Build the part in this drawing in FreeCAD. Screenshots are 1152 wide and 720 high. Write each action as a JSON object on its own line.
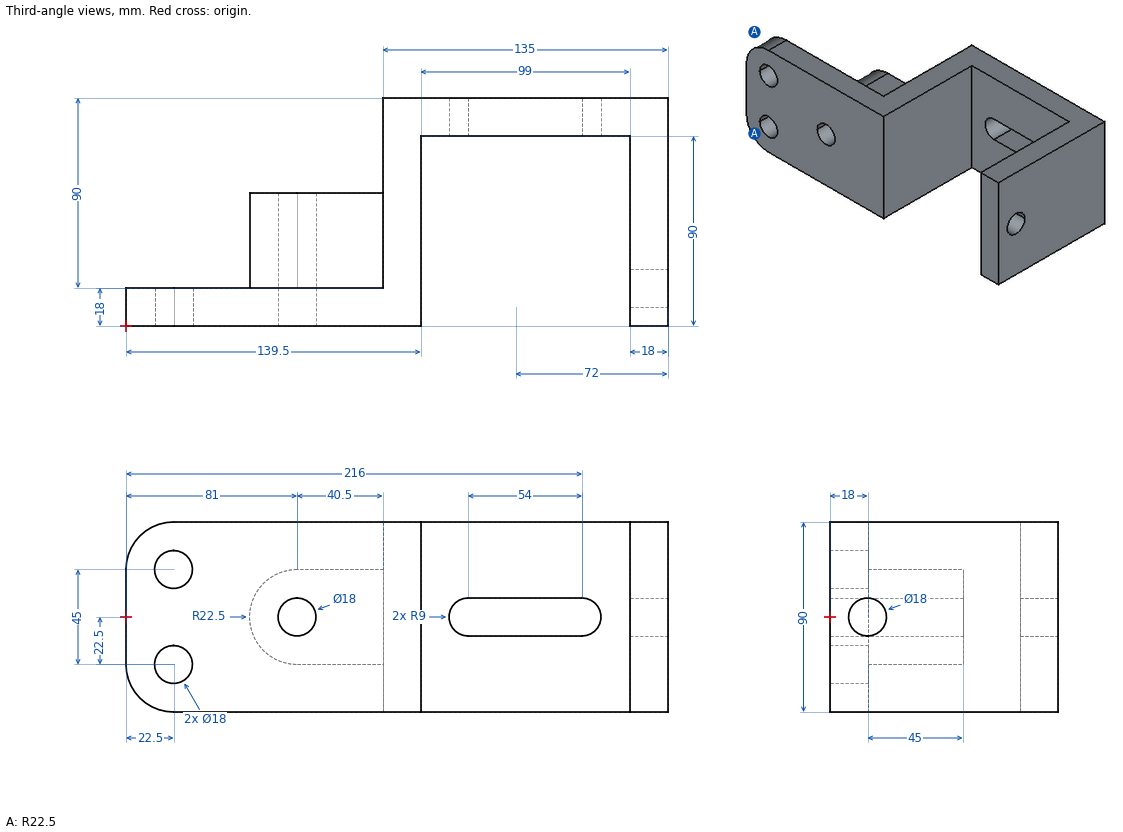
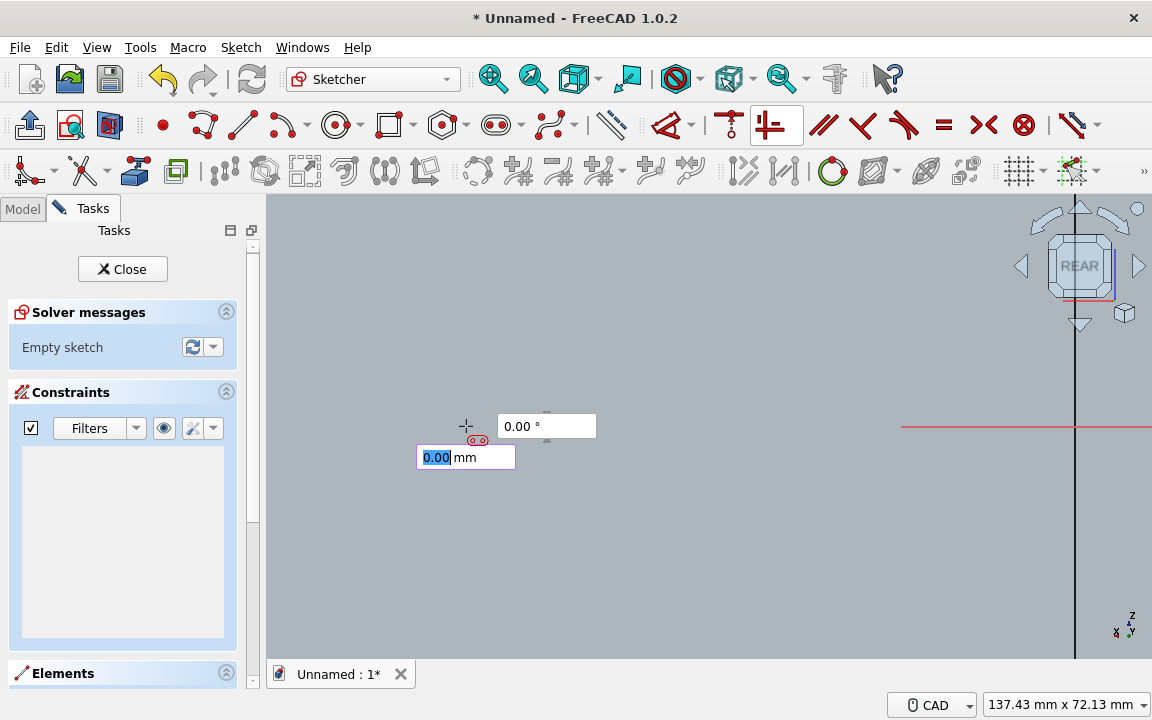
{"action": "left_click", "coordinate": [814, 417]}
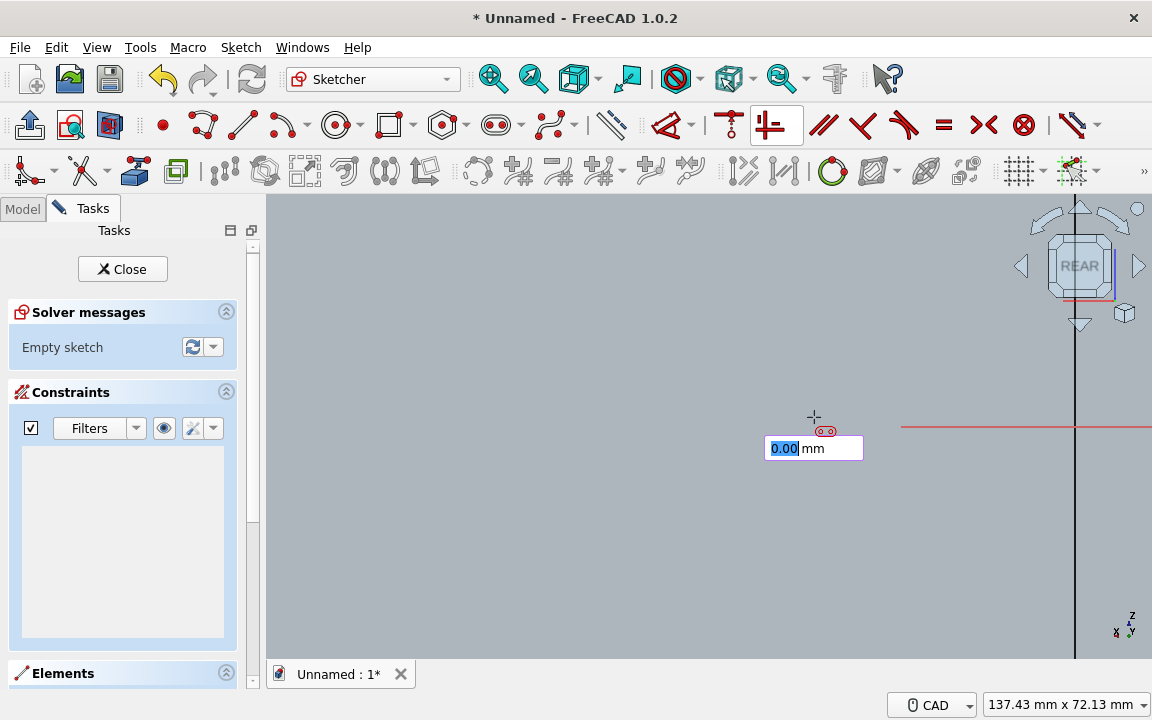
{"action": "left_click", "coordinate": [640, 485]}
{"action": "key", "text": "Escape"}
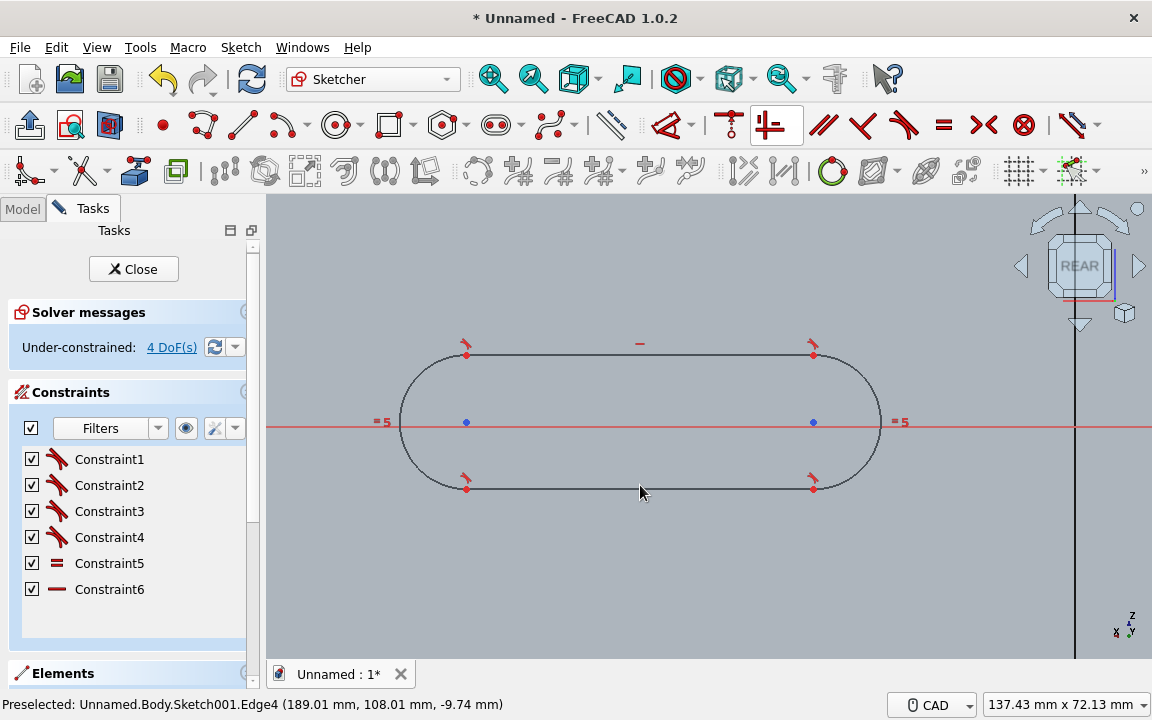
{"action": "left_click", "coordinate": [467, 422]}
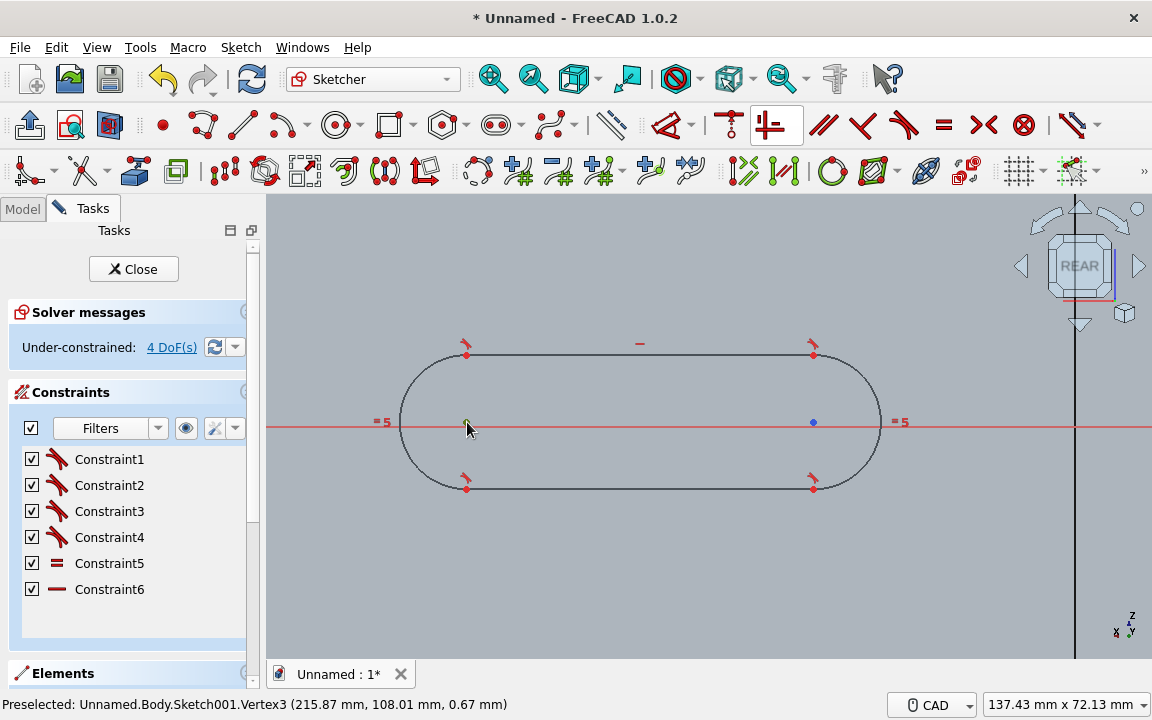
{"action": "left_click", "coordinate": [343, 426]}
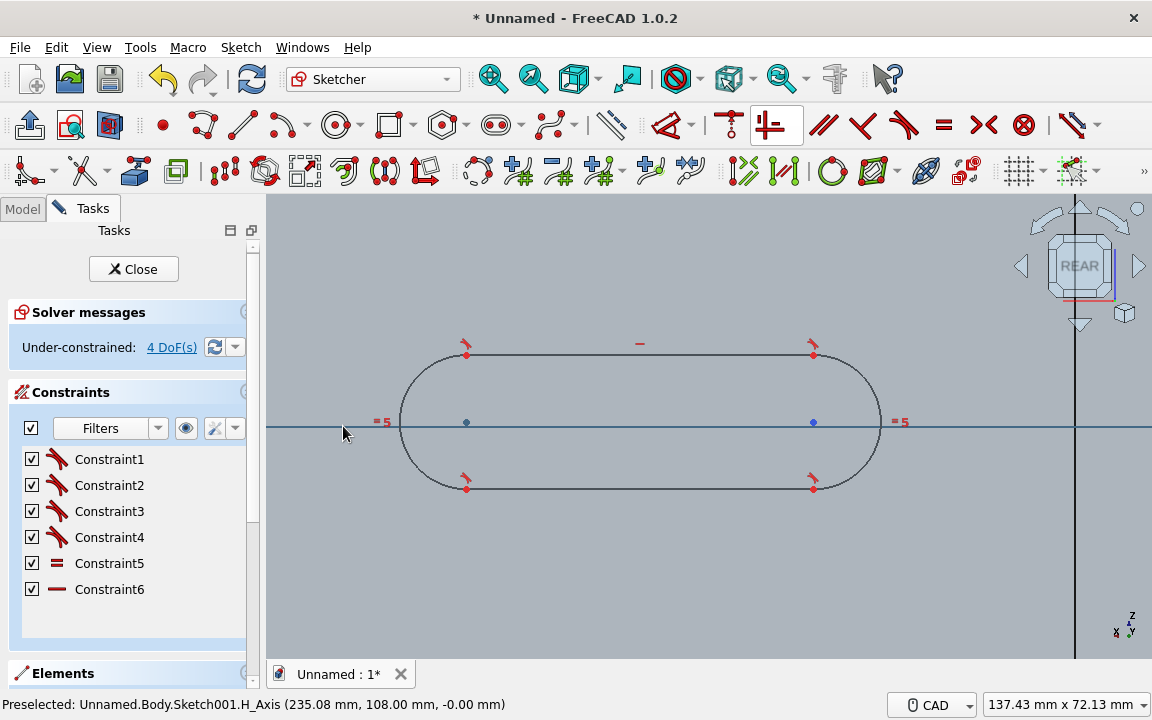
{"action": "left_click", "coordinate": [730, 126]}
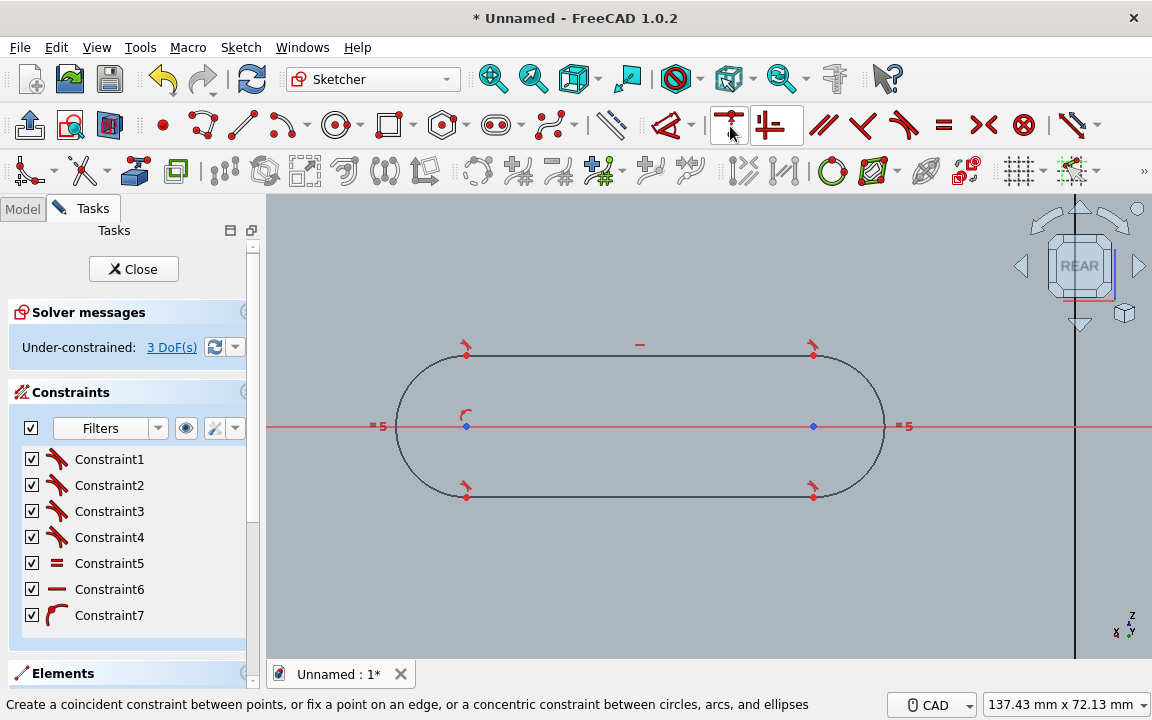
{"action": "left_click", "coordinate": [666, 126]}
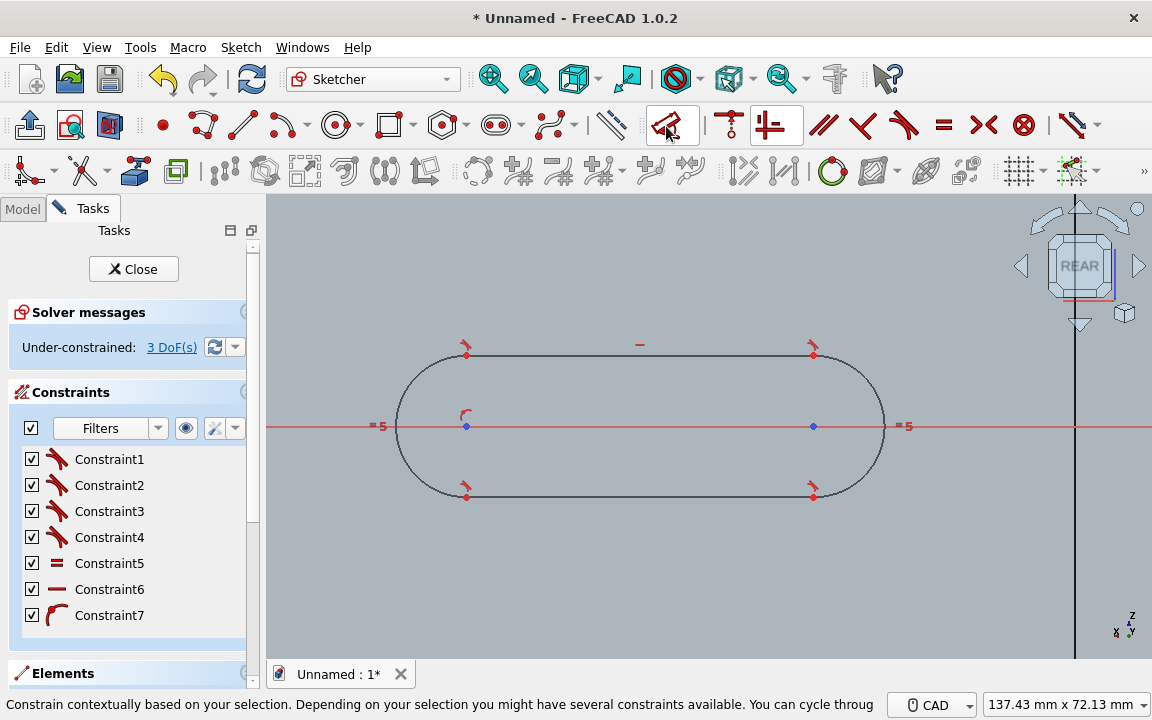
{"action": "left_click", "coordinate": [410, 385]}
{"action": "left_click", "coordinate": [384, 366]}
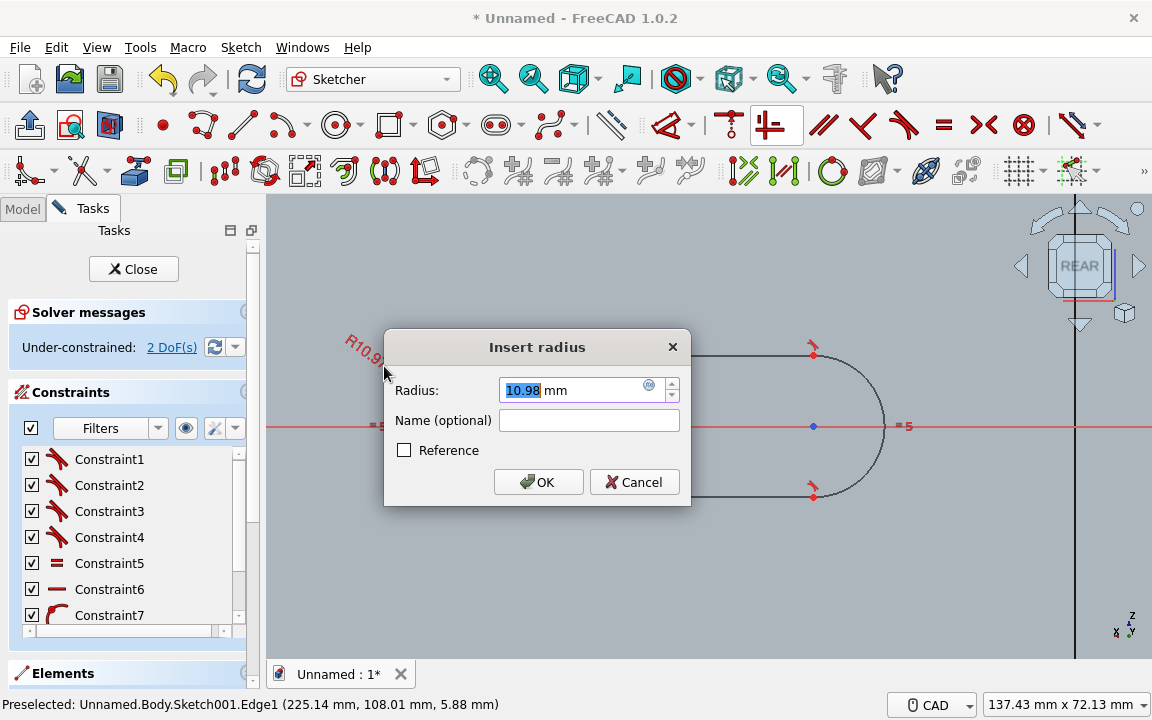
{"action": "type", "text": "9"}
{"action": "key", "text": "Return"}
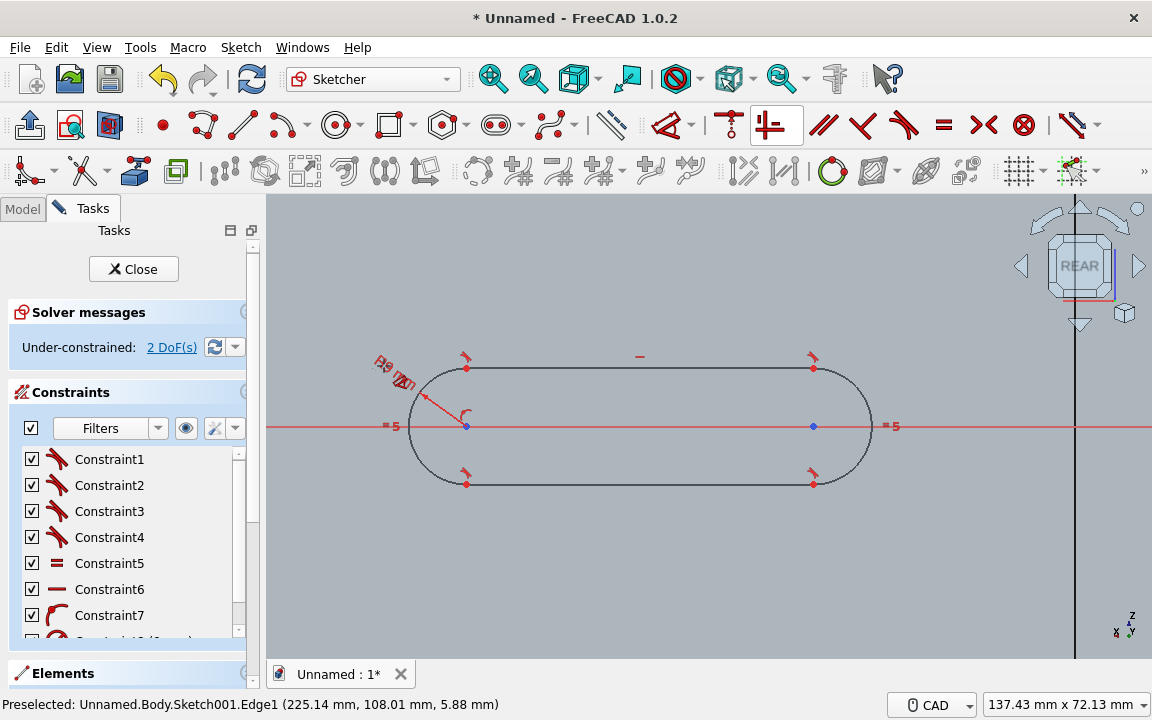
{"action": "left_click", "coordinate": [571, 368]}
{"action": "left_click", "coordinate": [640, 334]}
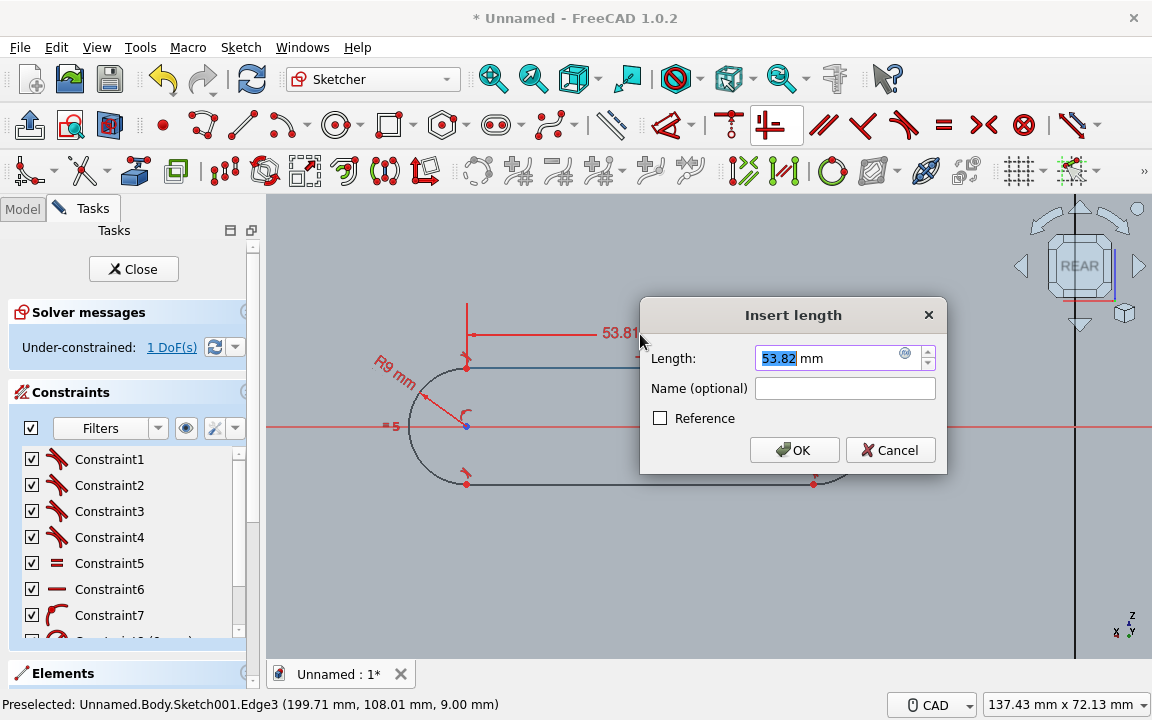
{"action": "type", "text": "54"}
{"action": "key", "text": "Return"}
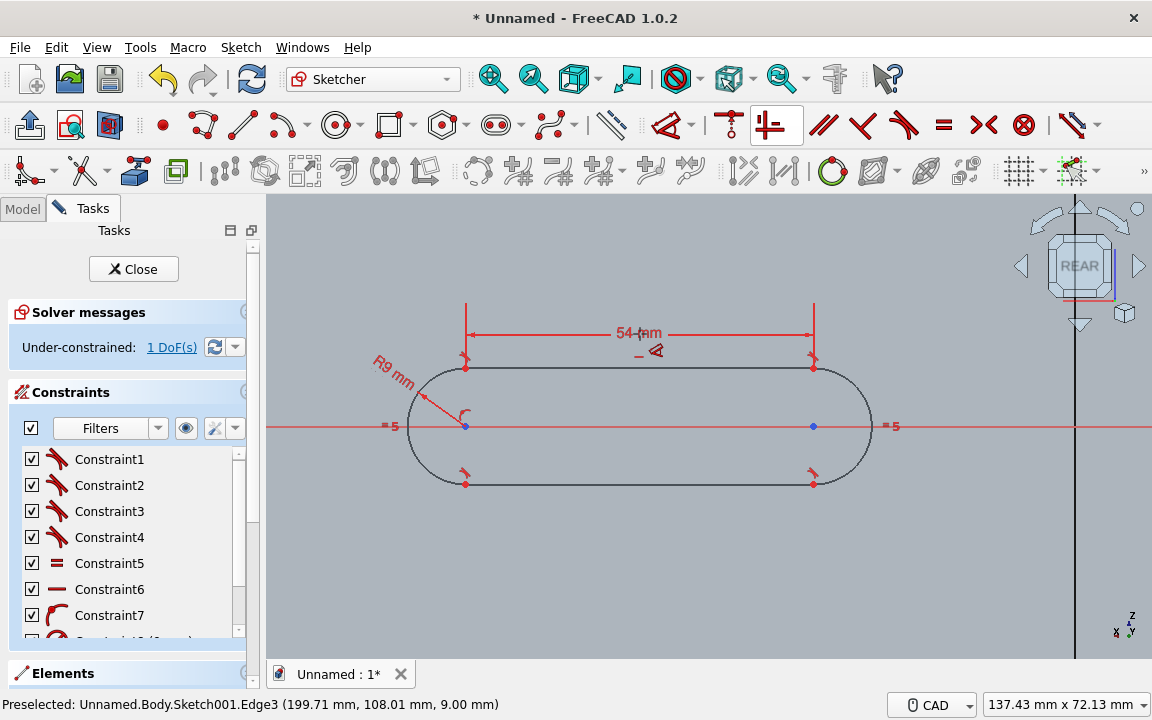
{"action": "left_click", "coordinate": [466, 368]}
{"action": "left_click", "coordinate": [726, 334]}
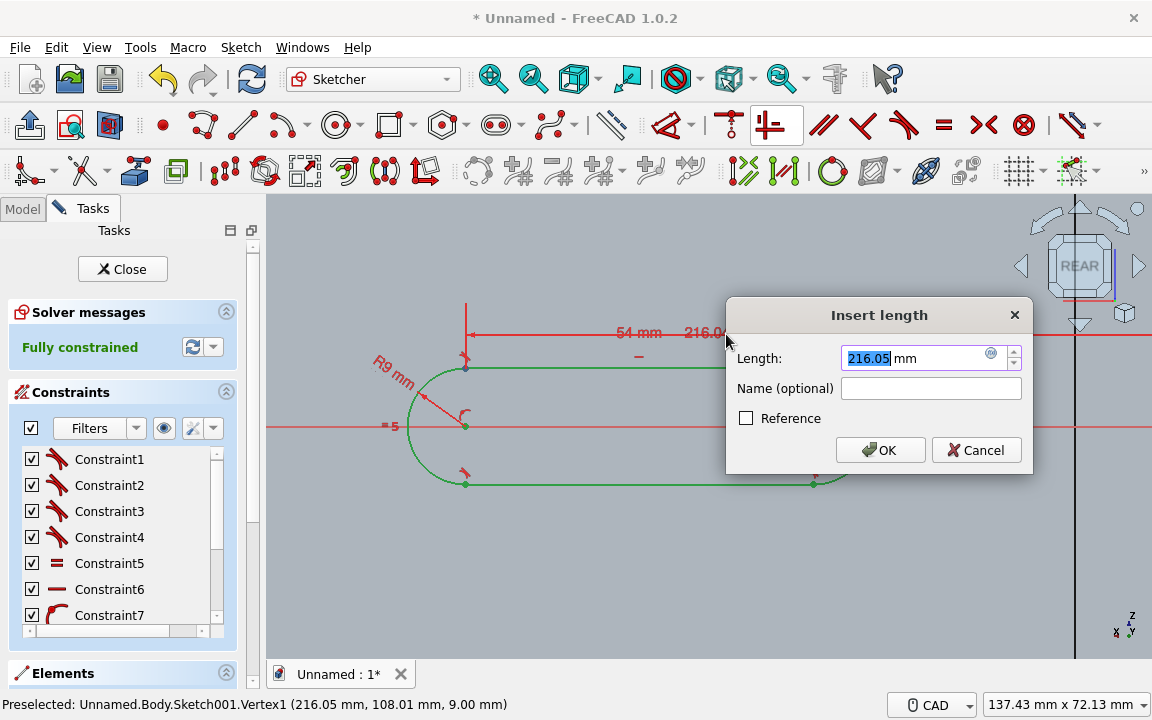
{"action": "type", "text": "216"}
{"action": "key", "text": "Return"}
{"action": "key", "text": "Escape"}